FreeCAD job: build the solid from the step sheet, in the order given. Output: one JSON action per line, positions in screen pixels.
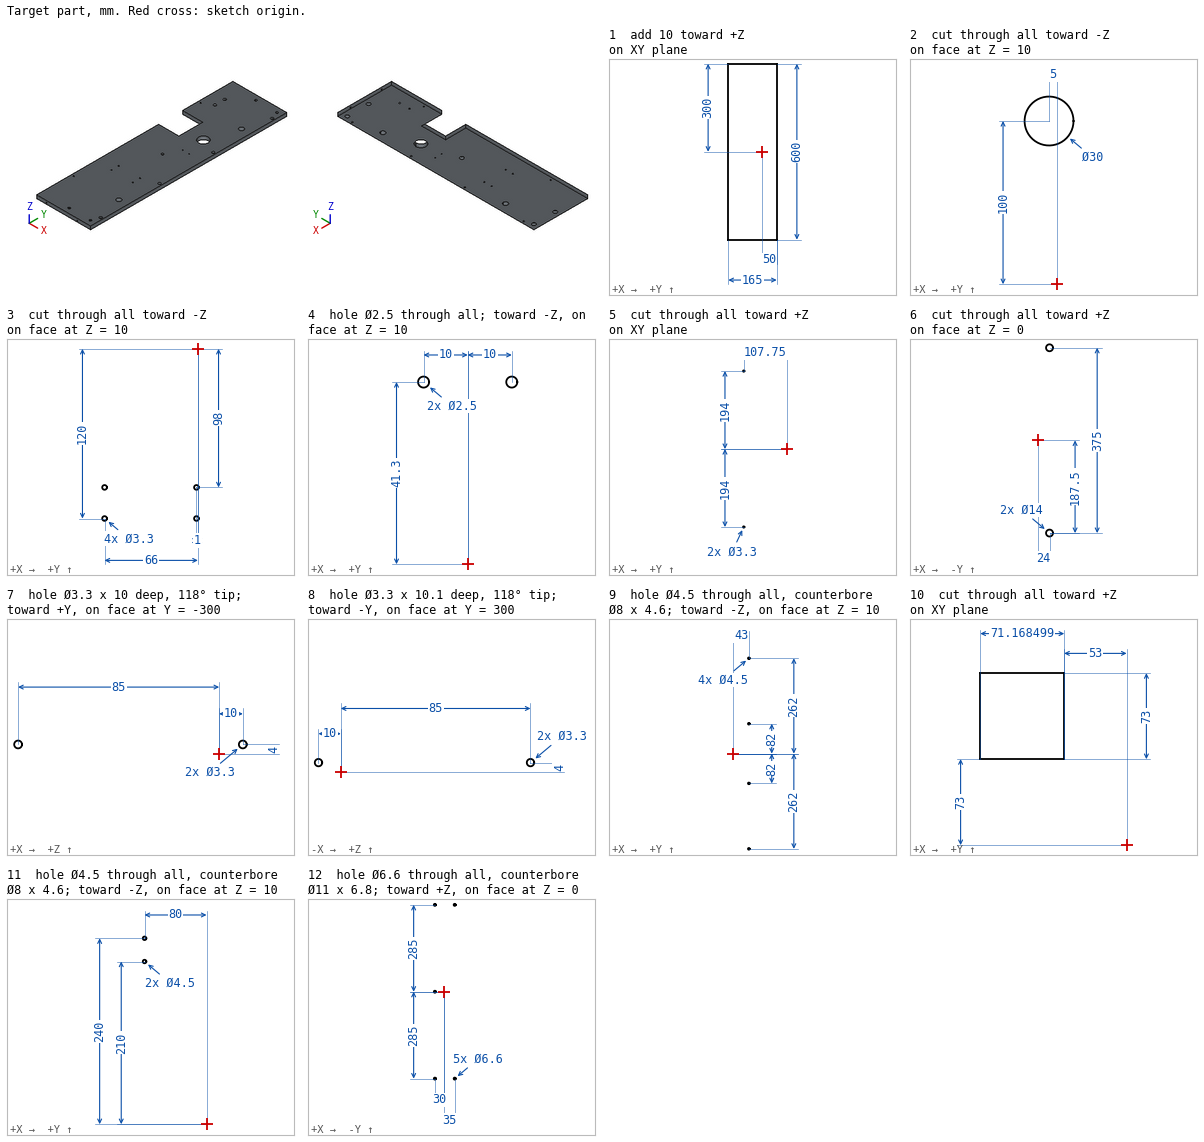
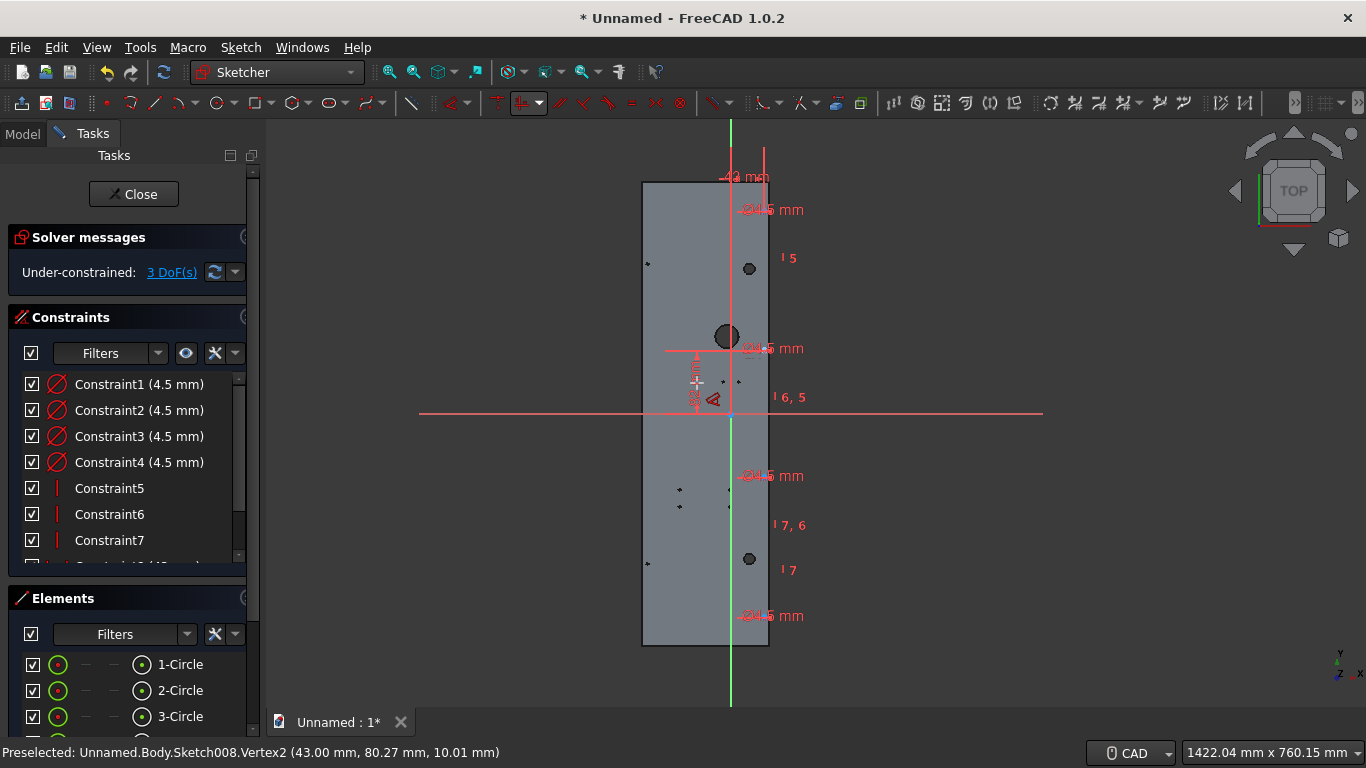
{"action": "left_click", "coordinate": [764, 478]}
{"action": "left_click", "coordinate": [697, 446]}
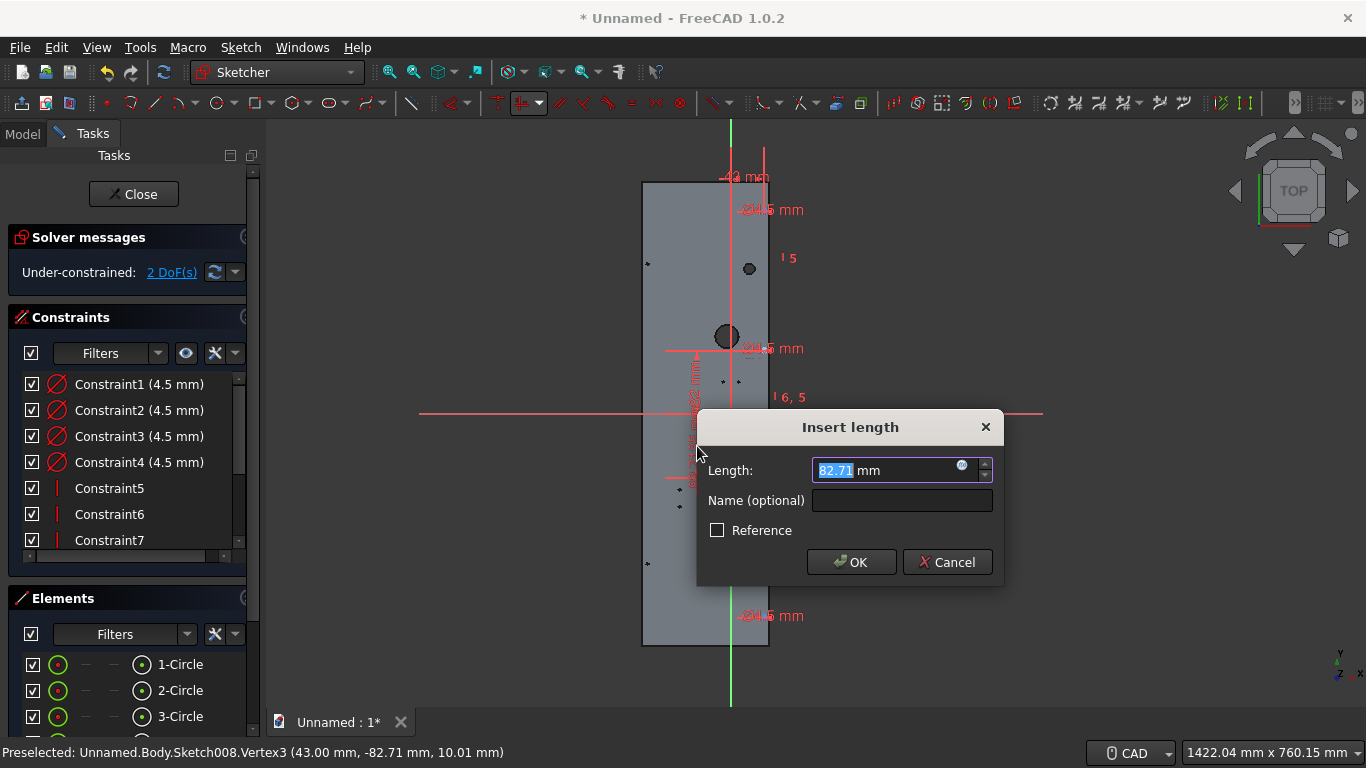
{"action": "type", "text": "82"}
{"action": "key", "text": "Return"}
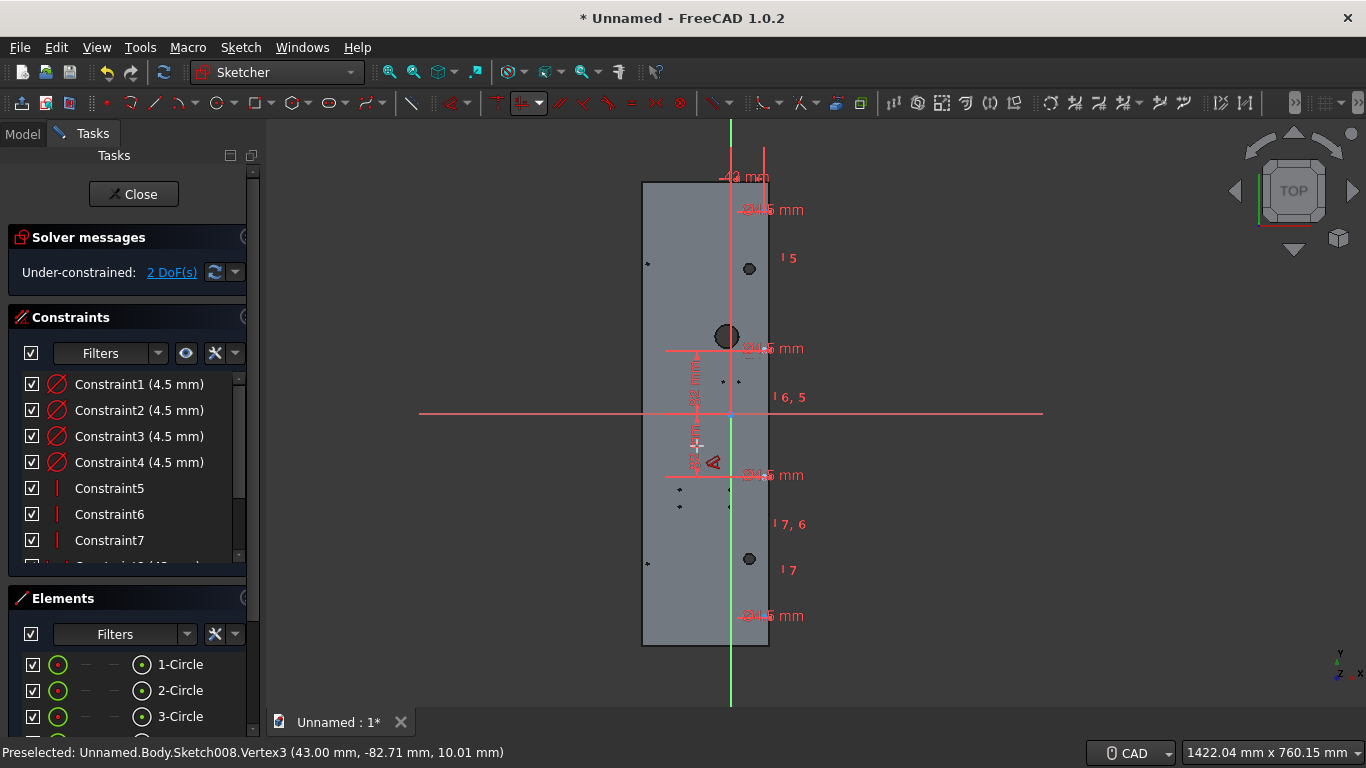
{"action": "left_click", "coordinate": [764, 212]}
{"action": "left_click", "coordinate": [697, 313]}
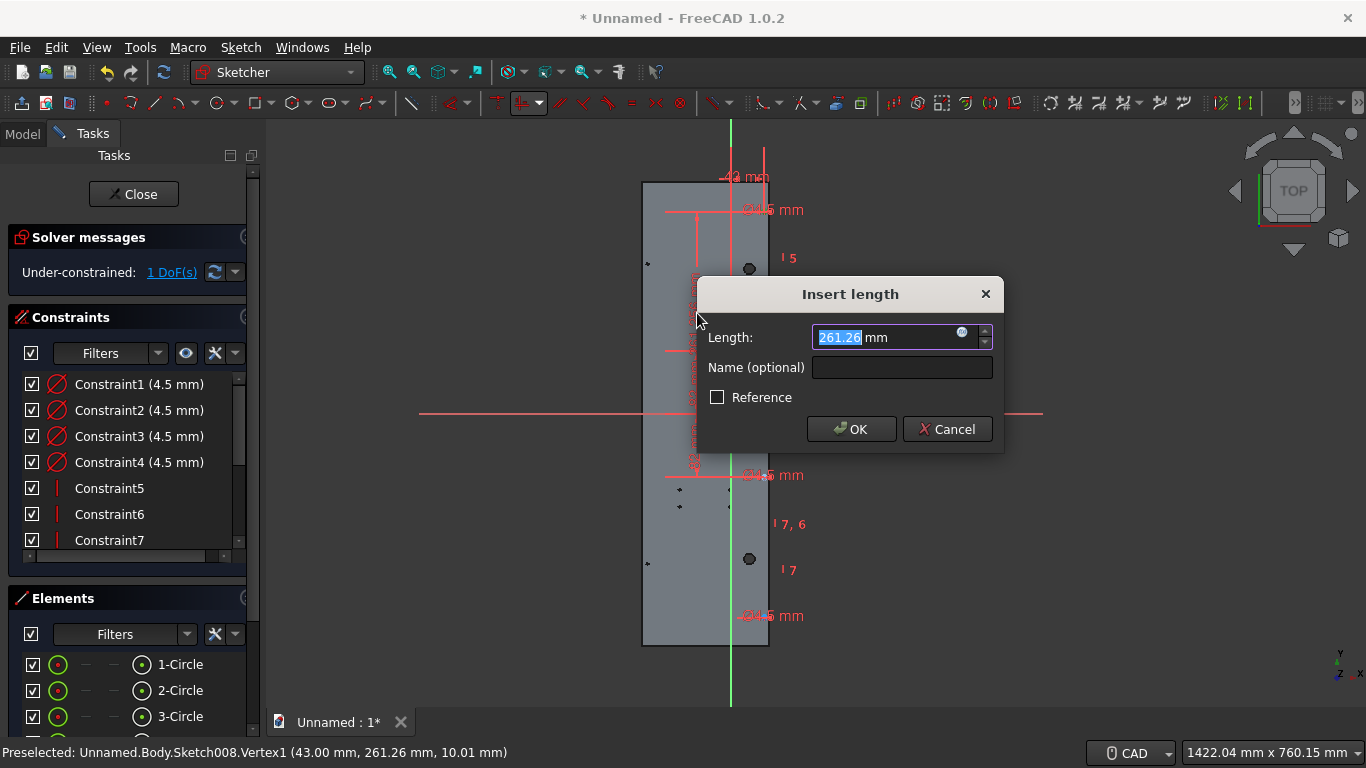
{"action": "type", "text": "262"}
{"action": "key", "text": "Return"}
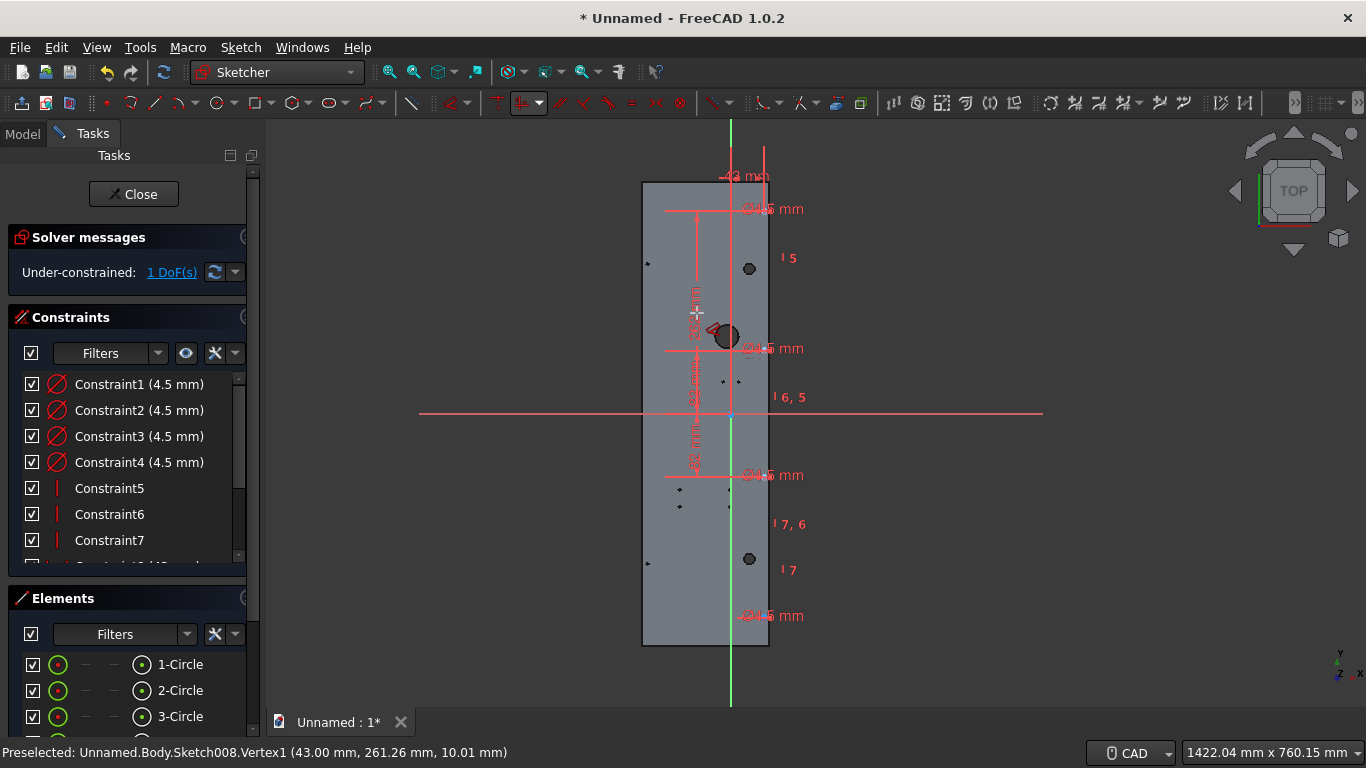
{"action": "left_click", "coordinate": [764, 618]}
{"action": "left_click", "coordinate": [697, 516]}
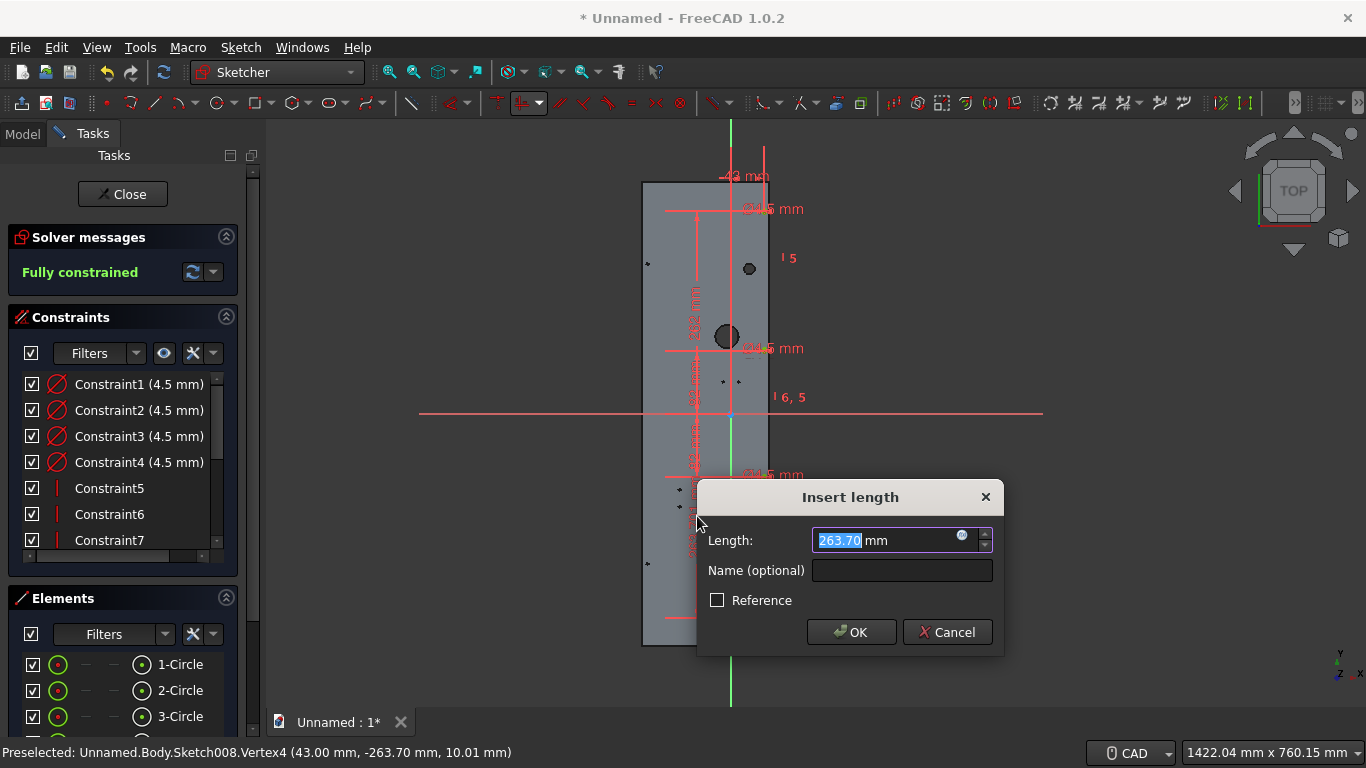
{"action": "type", "text": "262"}
{"action": "key", "text": "Return"}
{"action": "key", "text": "Escape"}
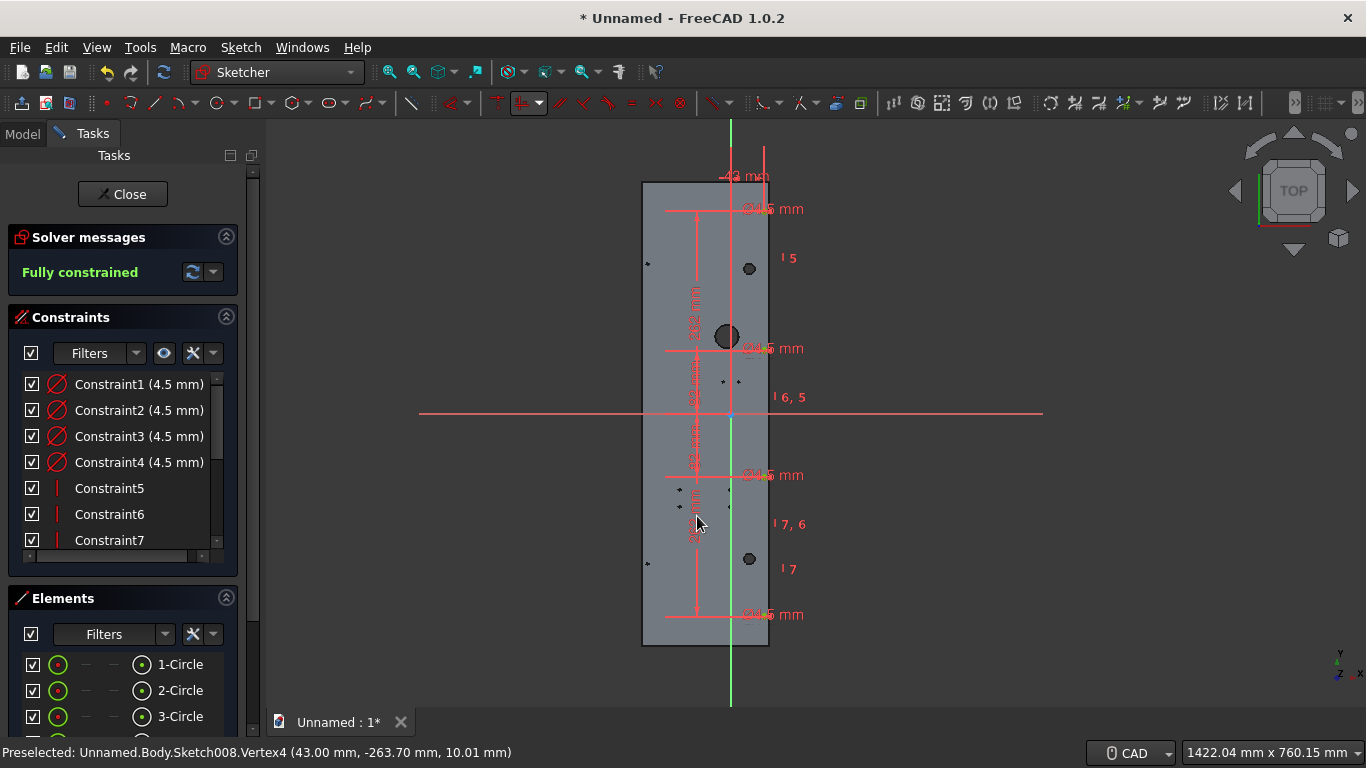
{"action": "left_click", "coordinate": [123, 194]}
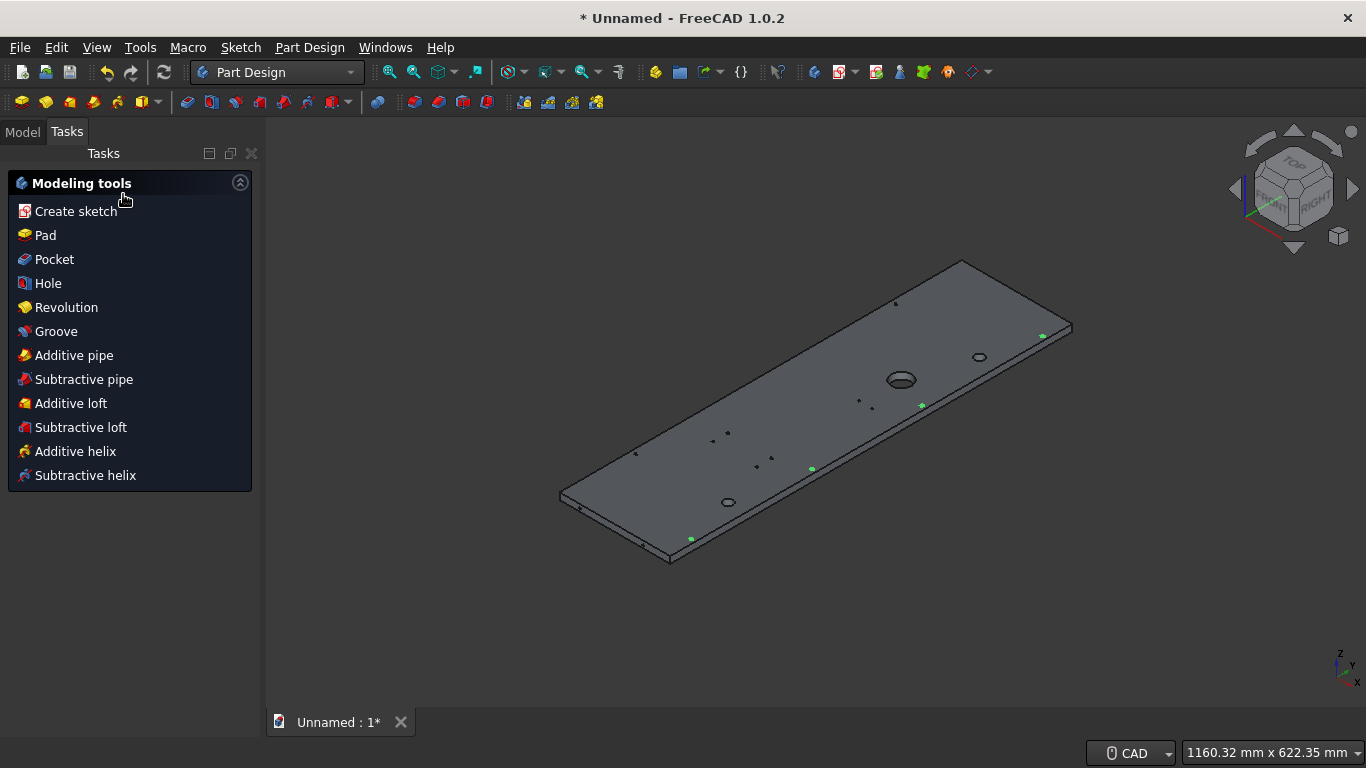
{"action": "left_click", "coordinate": [212, 102]}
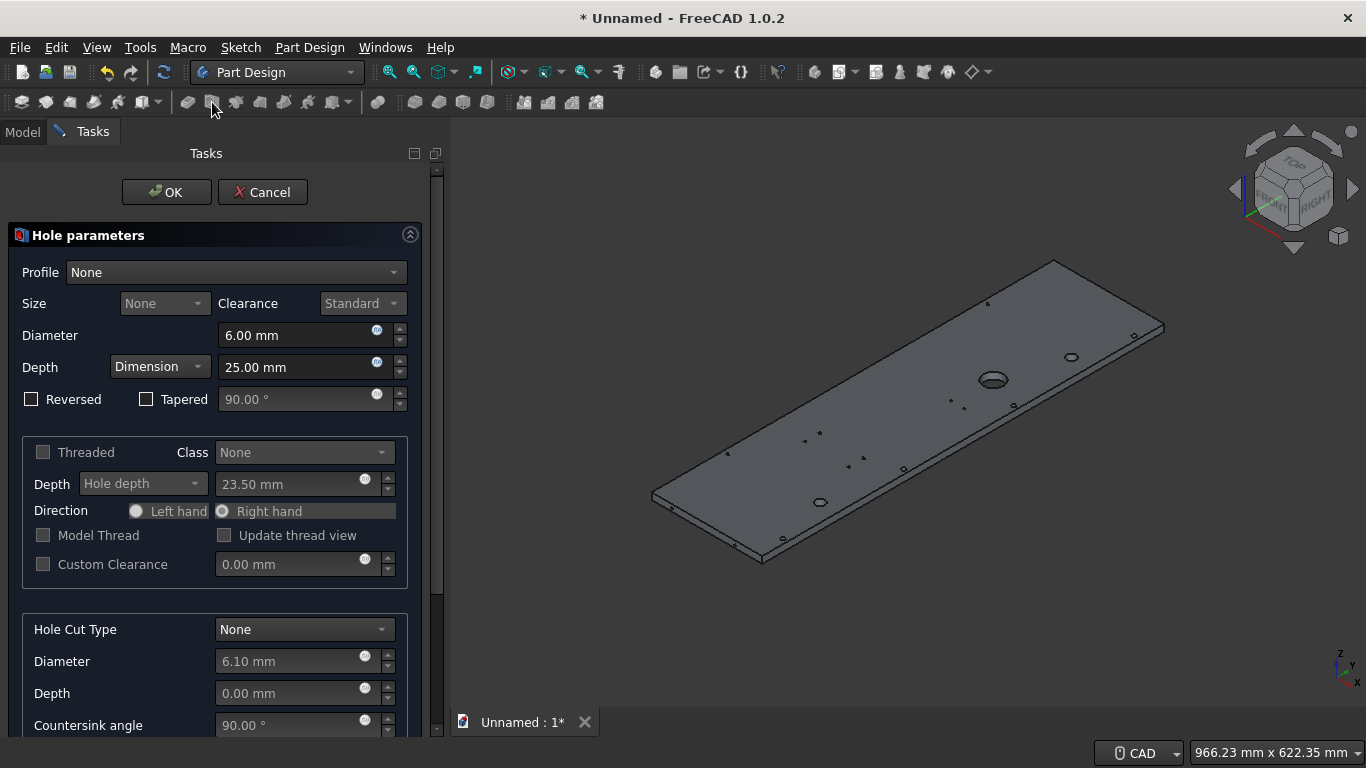
{"action": "triple_click", "coordinate": [305, 335]}